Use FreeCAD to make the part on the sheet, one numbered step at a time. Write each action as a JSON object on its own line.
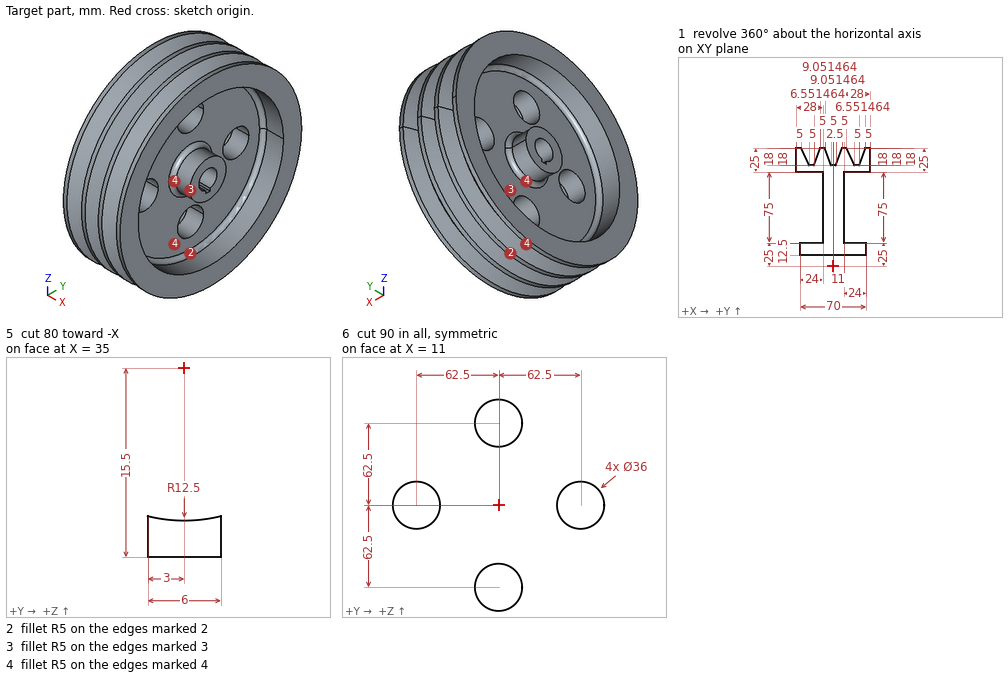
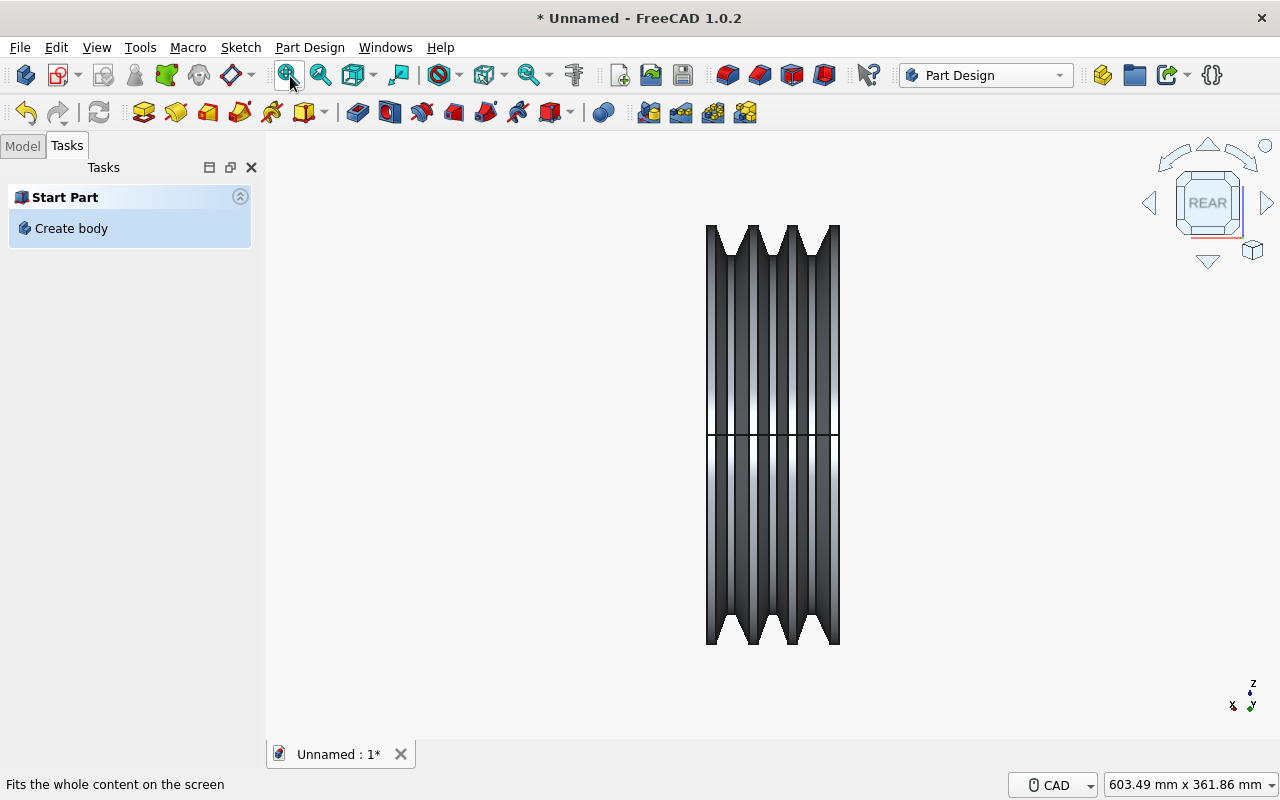
{"action": "key", "text": "6"}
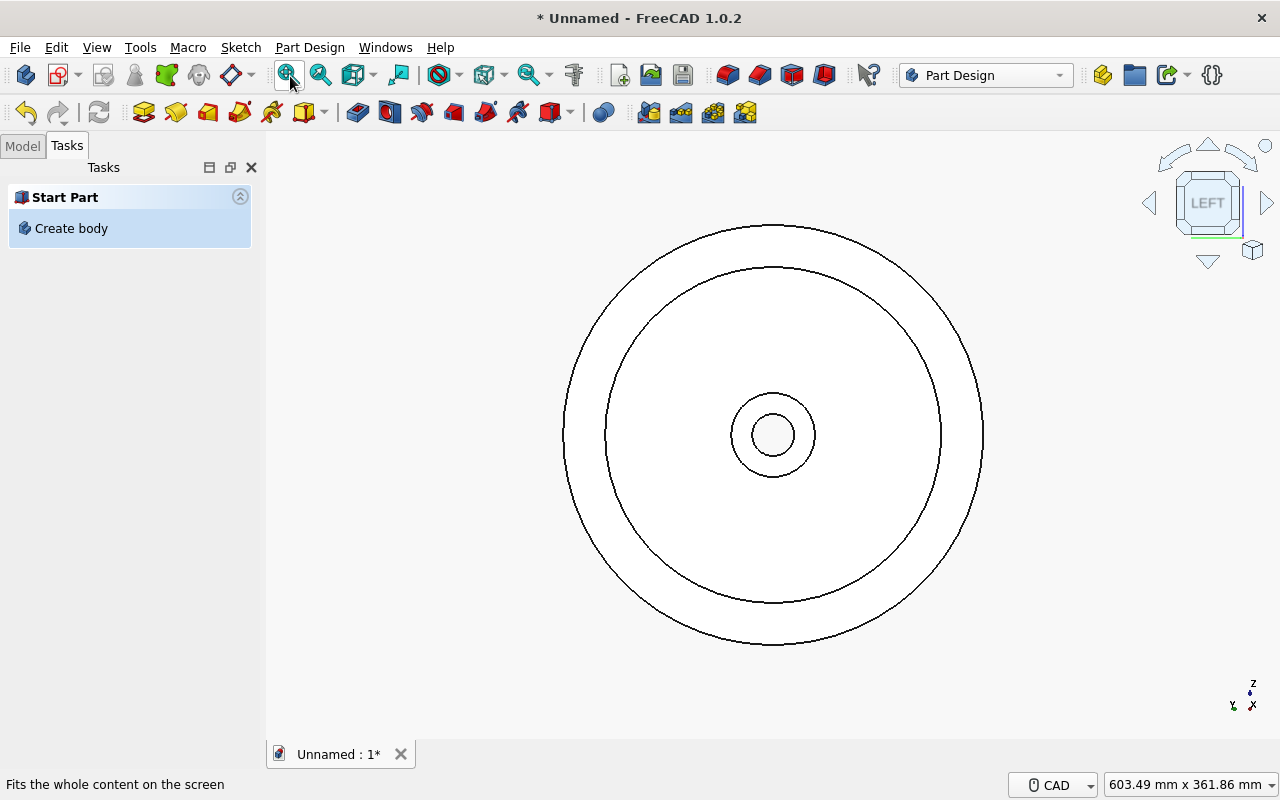
{"action": "key", "text": "v 3"}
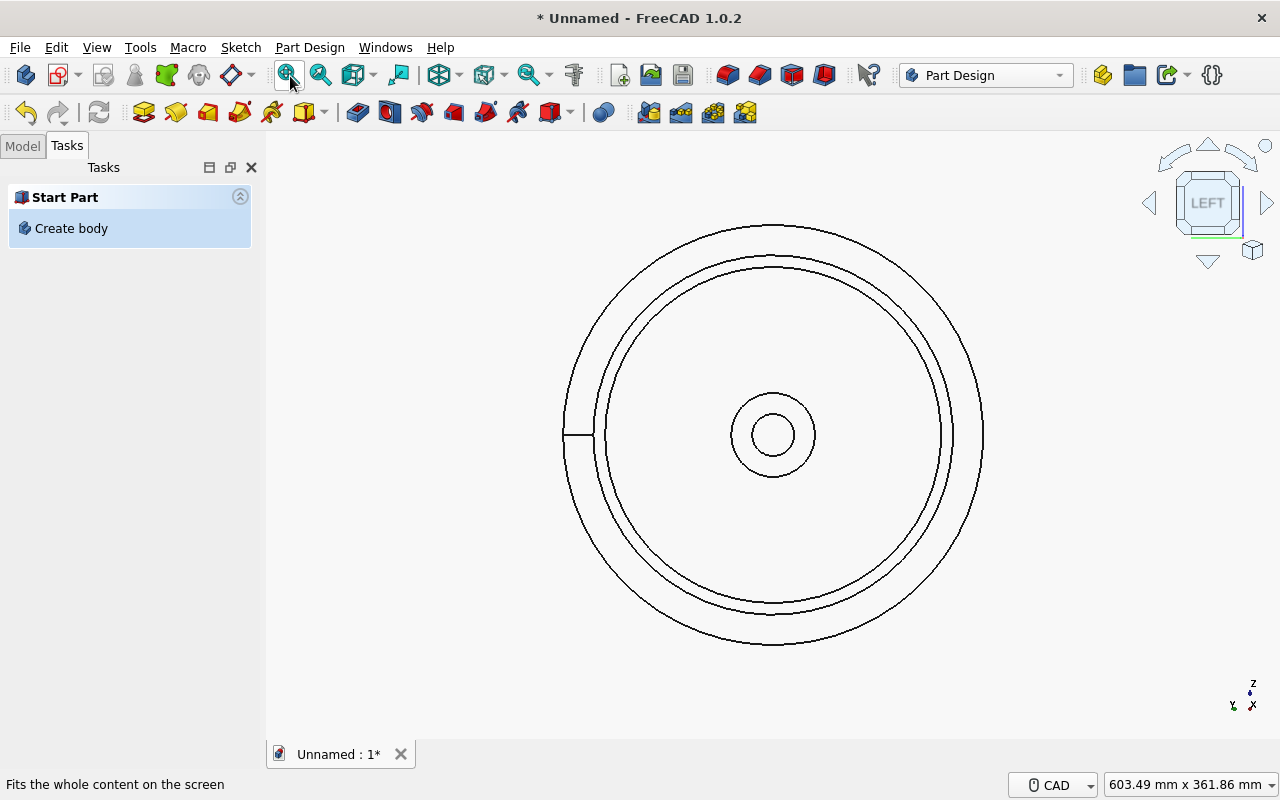
{"action": "key", "text": "0"}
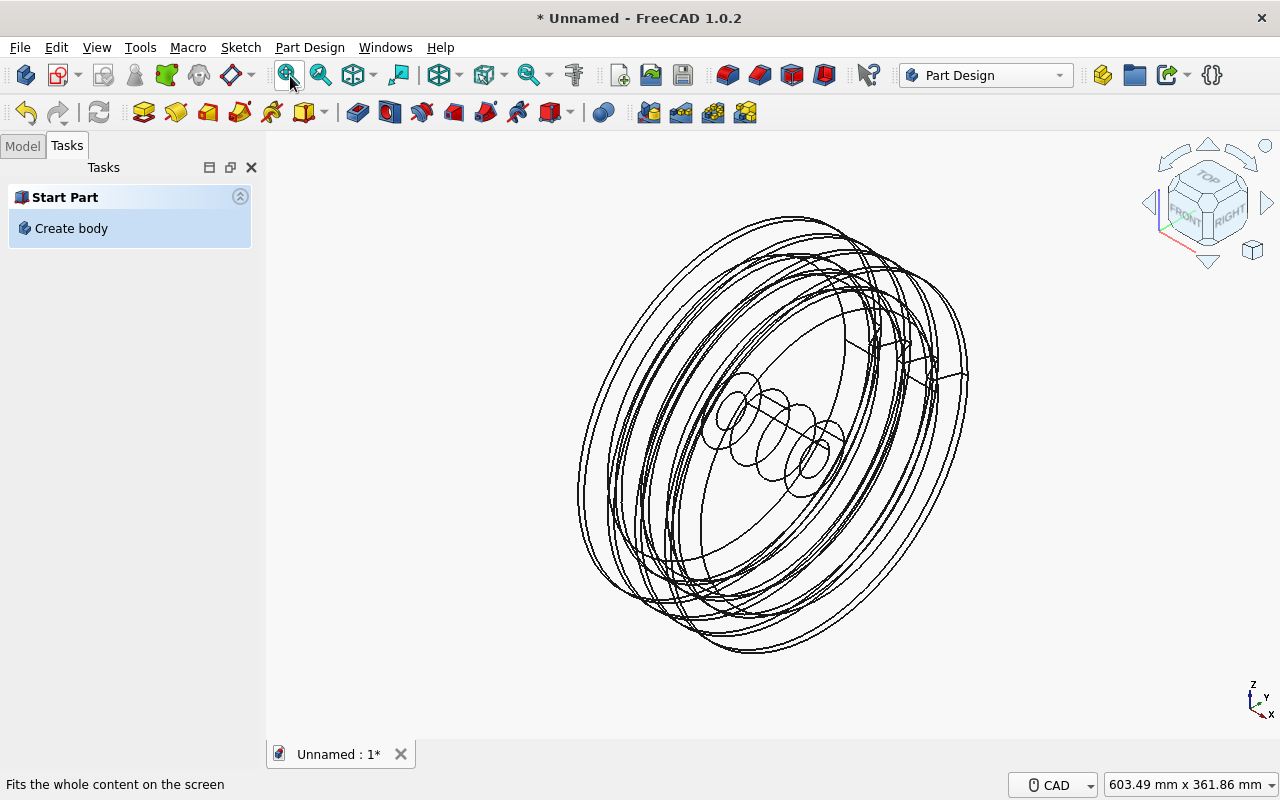
{"action": "left_click", "coordinate": [690, 416]}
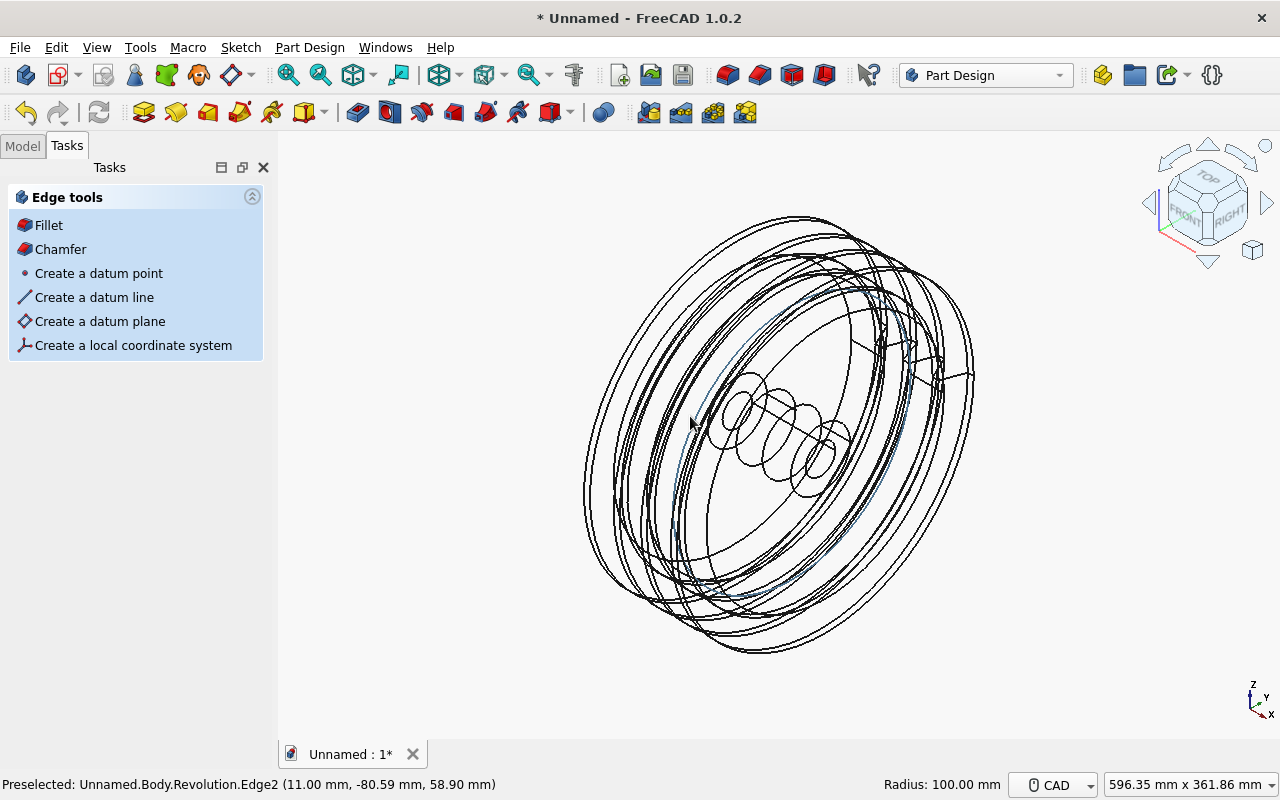
{"action": "key", "text": "v 1"}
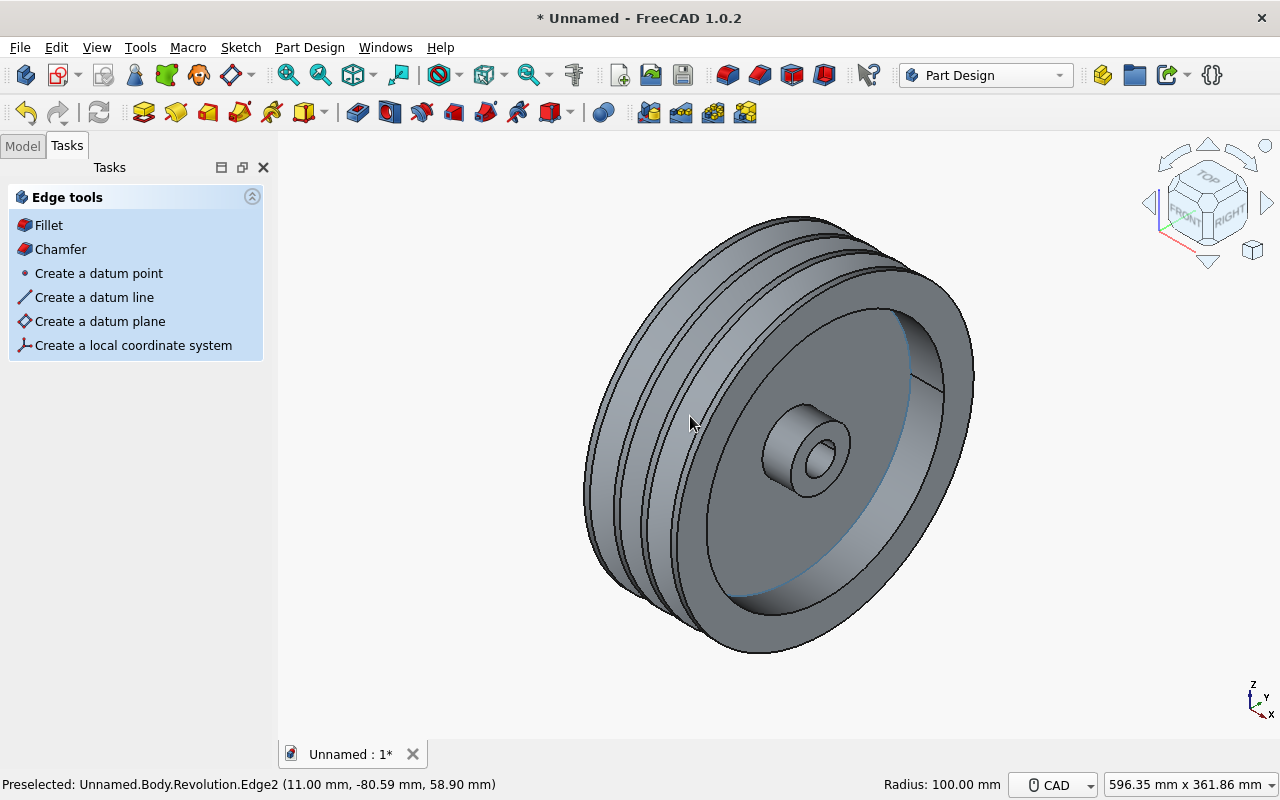
{"action": "left_click", "coordinate": [728, 76]}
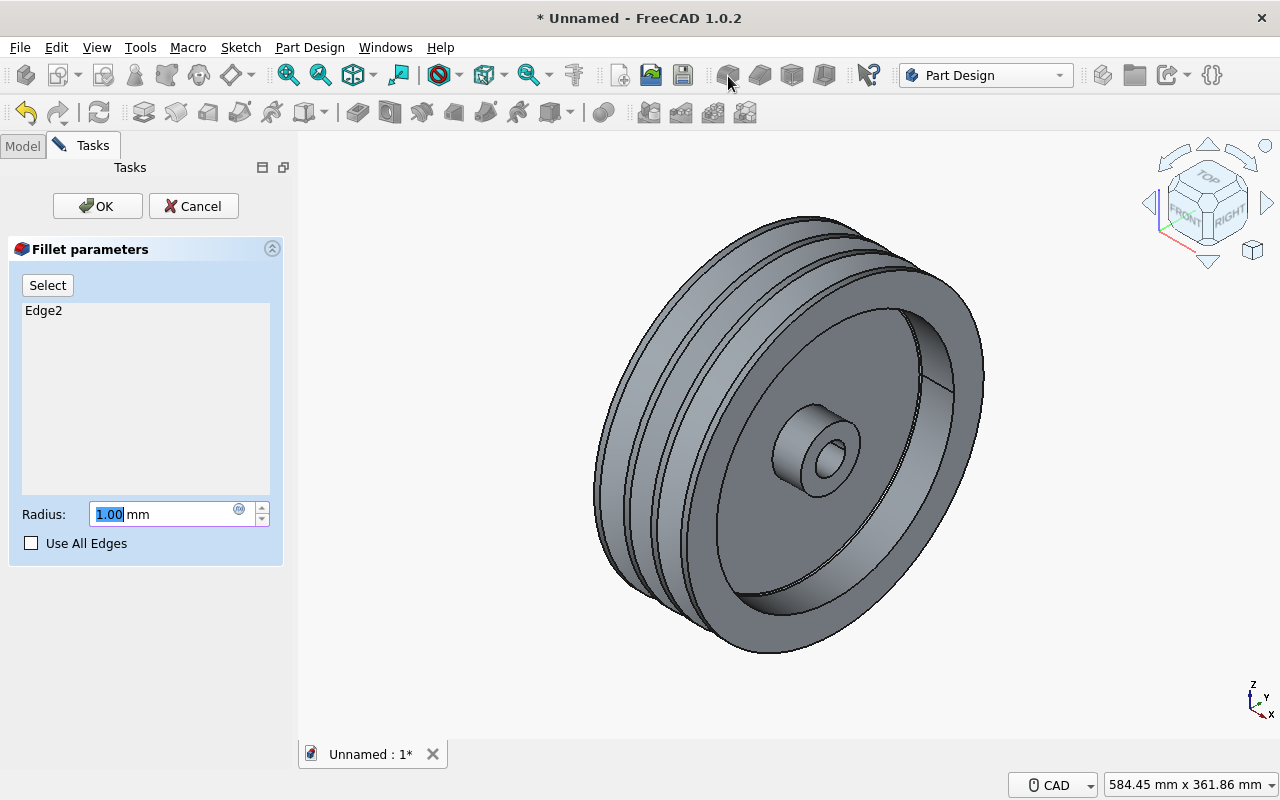
{"action": "type", "text": "5"}
{"action": "key", "text": "Tab"}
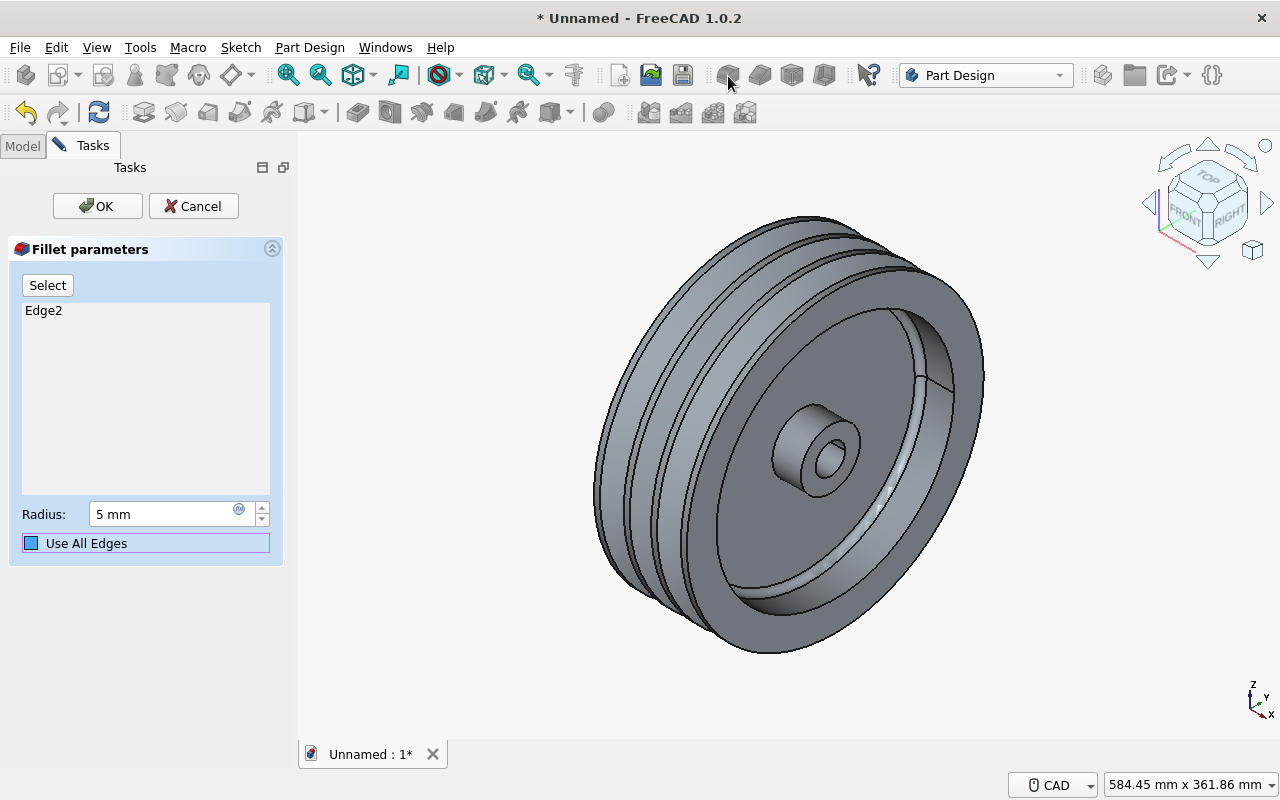
{"action": "left_click", "coordinate": [98, 206]}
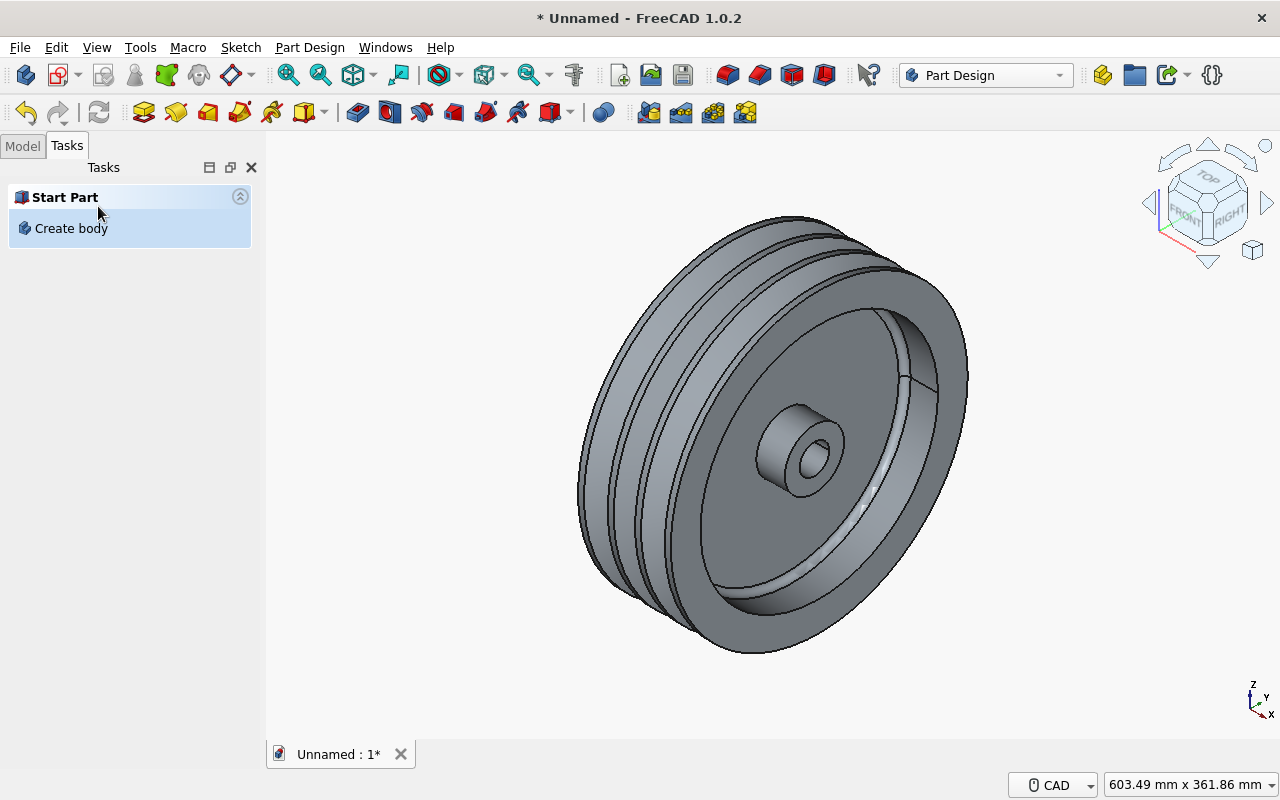
{"action": "key", "text": "2"}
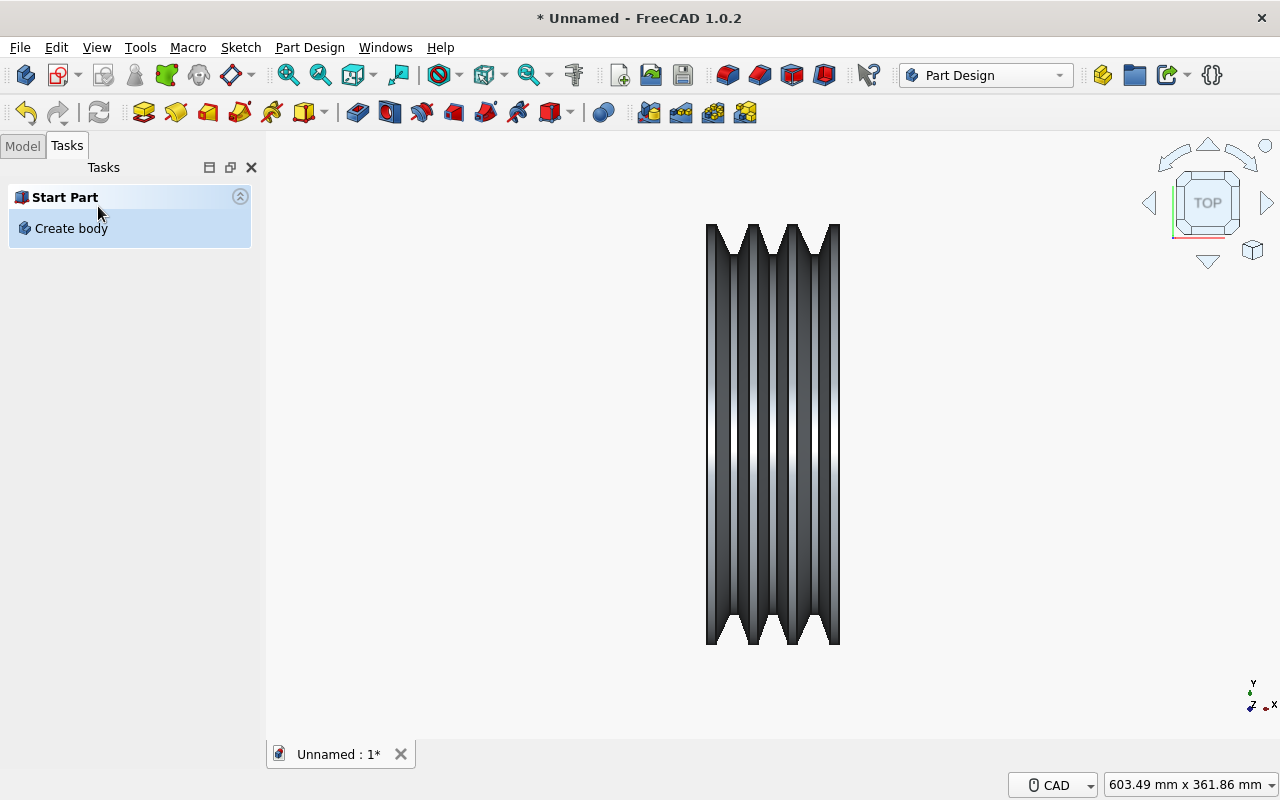
{"action": "key", "text": "0"}